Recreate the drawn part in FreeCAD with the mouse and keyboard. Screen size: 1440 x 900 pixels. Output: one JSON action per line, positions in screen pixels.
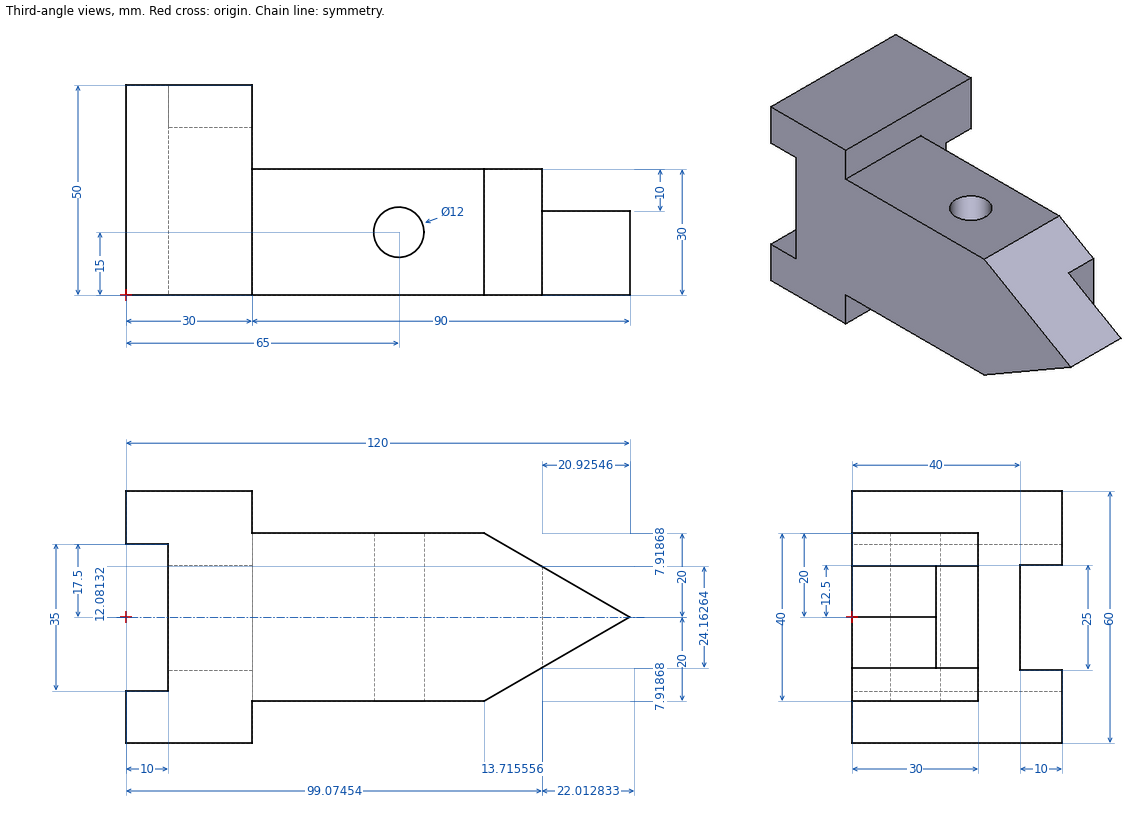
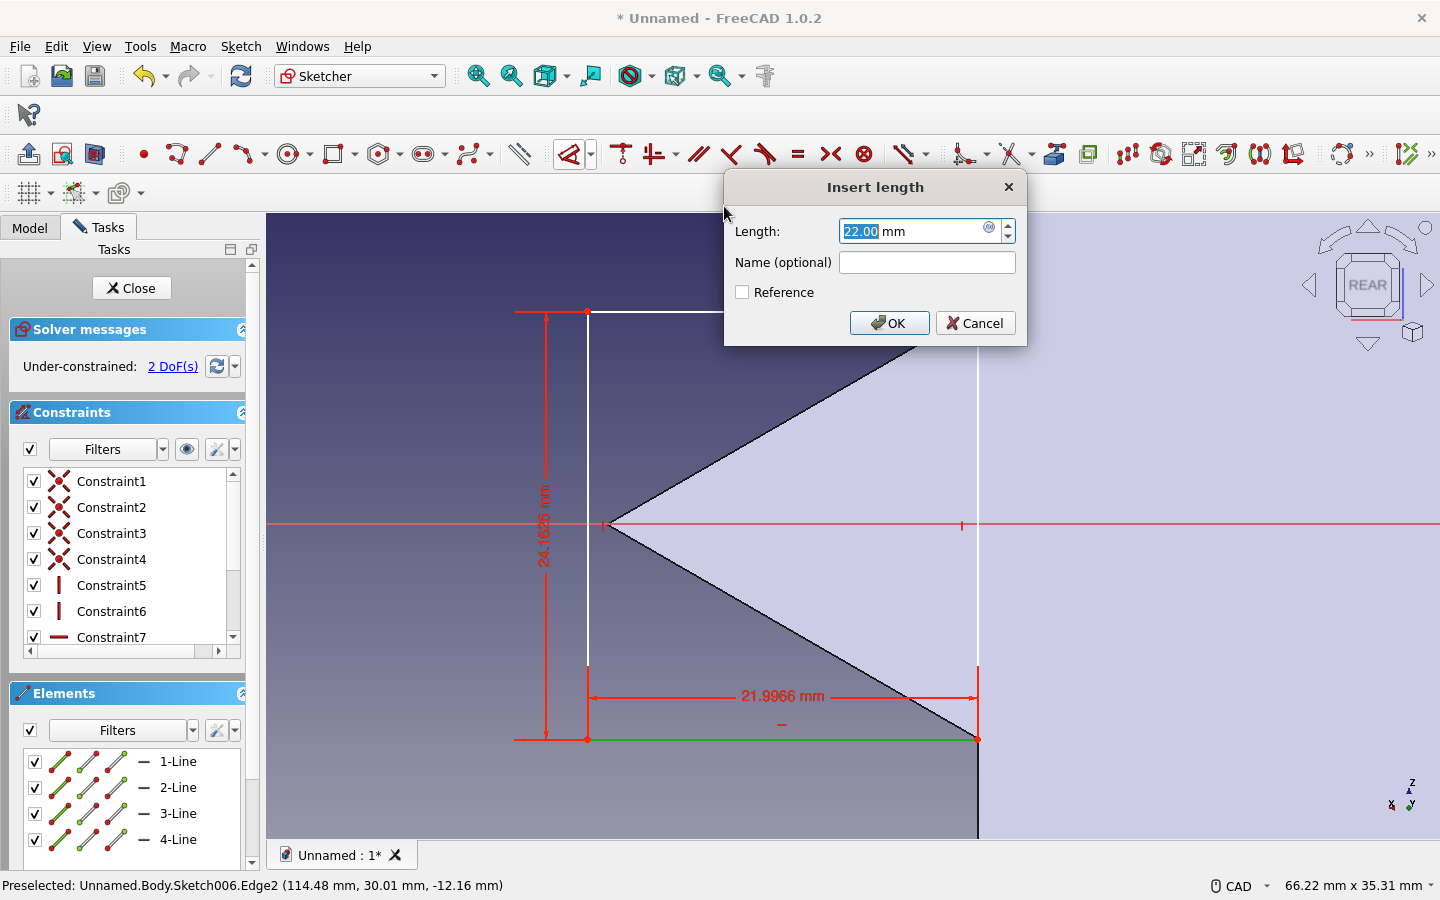
{"action": "type", "text": "22.012833"}
{"action": "key", "text": "Return"}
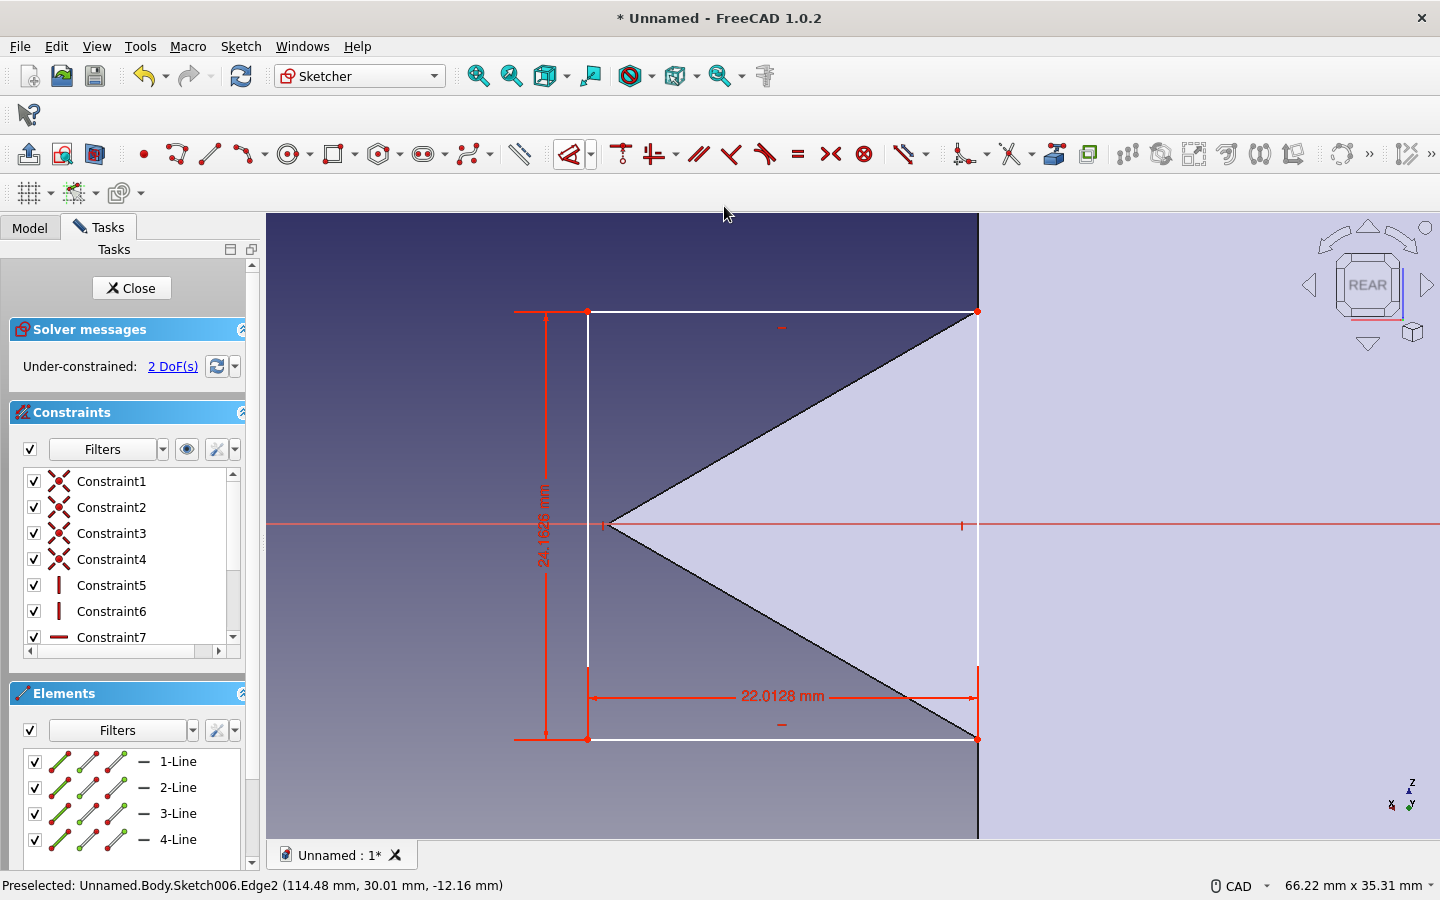
{"action": "left_click", "coordinate": [588, 312]}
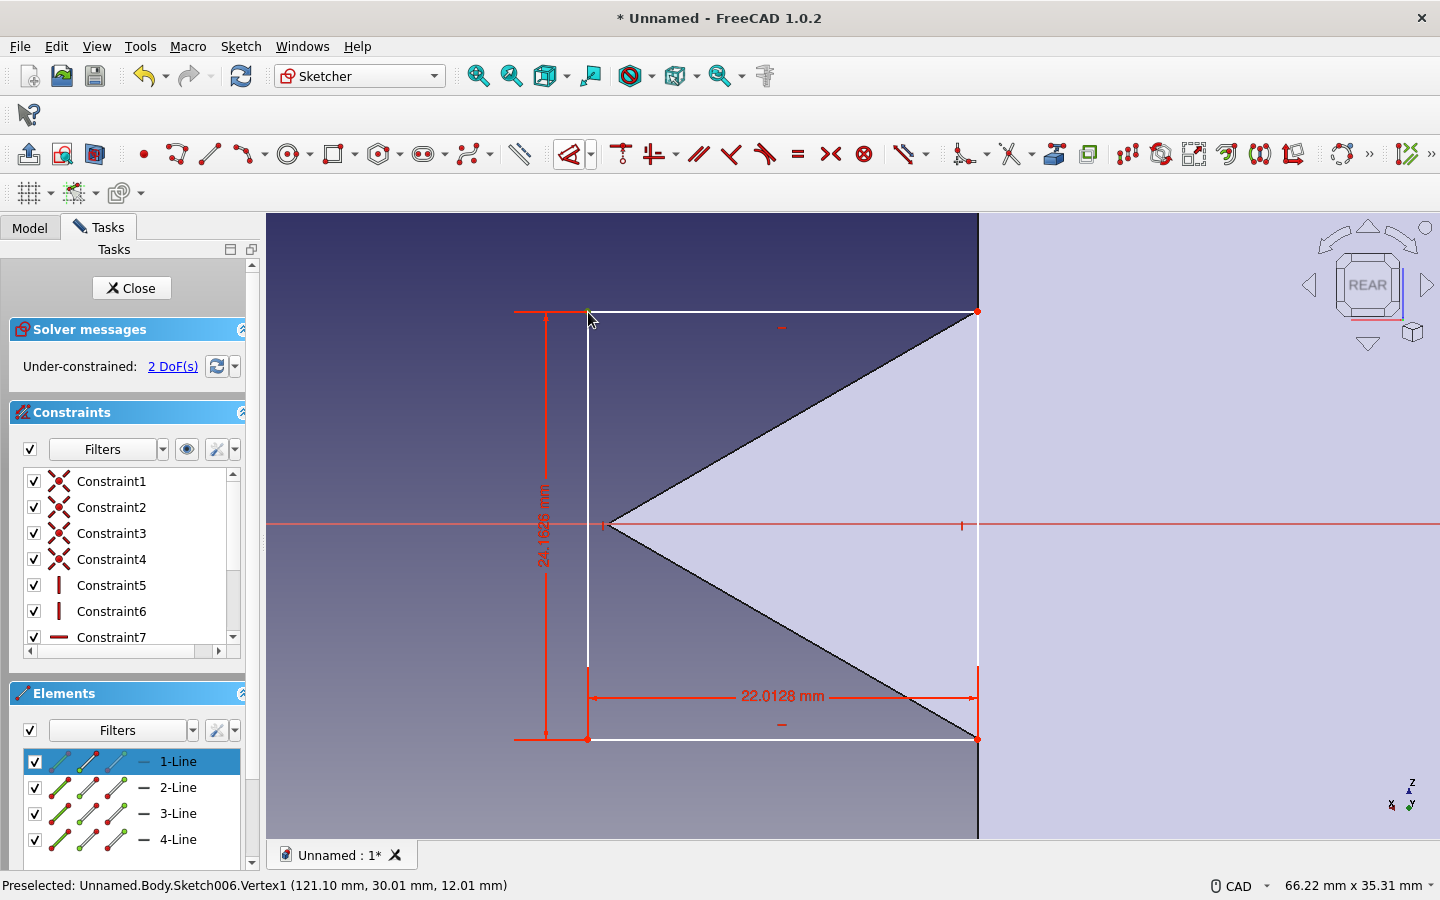
{"action": "left_click", "coordinate": [590, 154]}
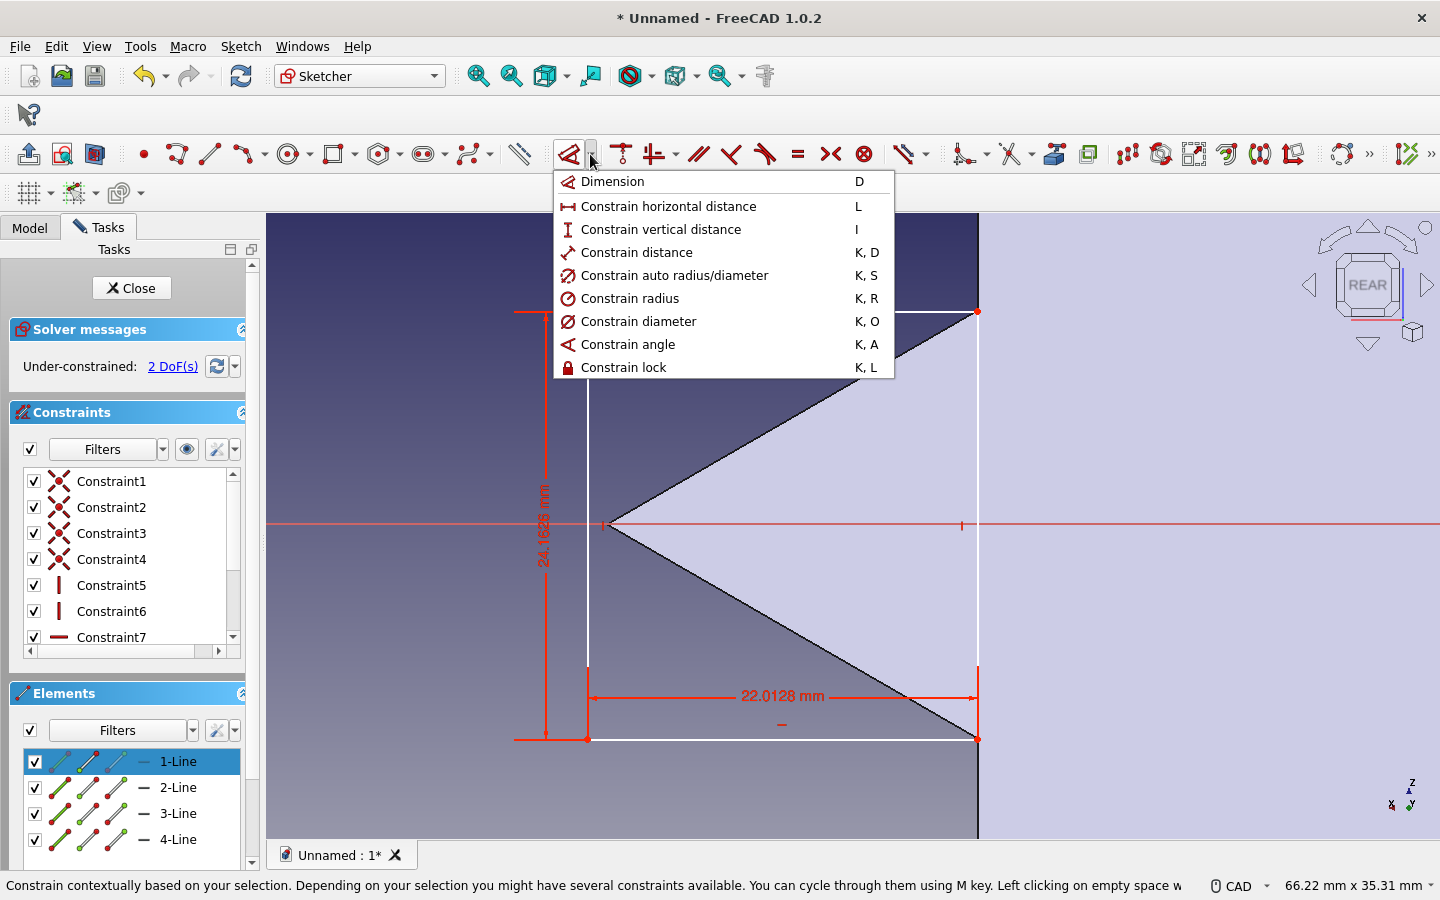
{"action": "left_click", "coordinate": [724, 230]}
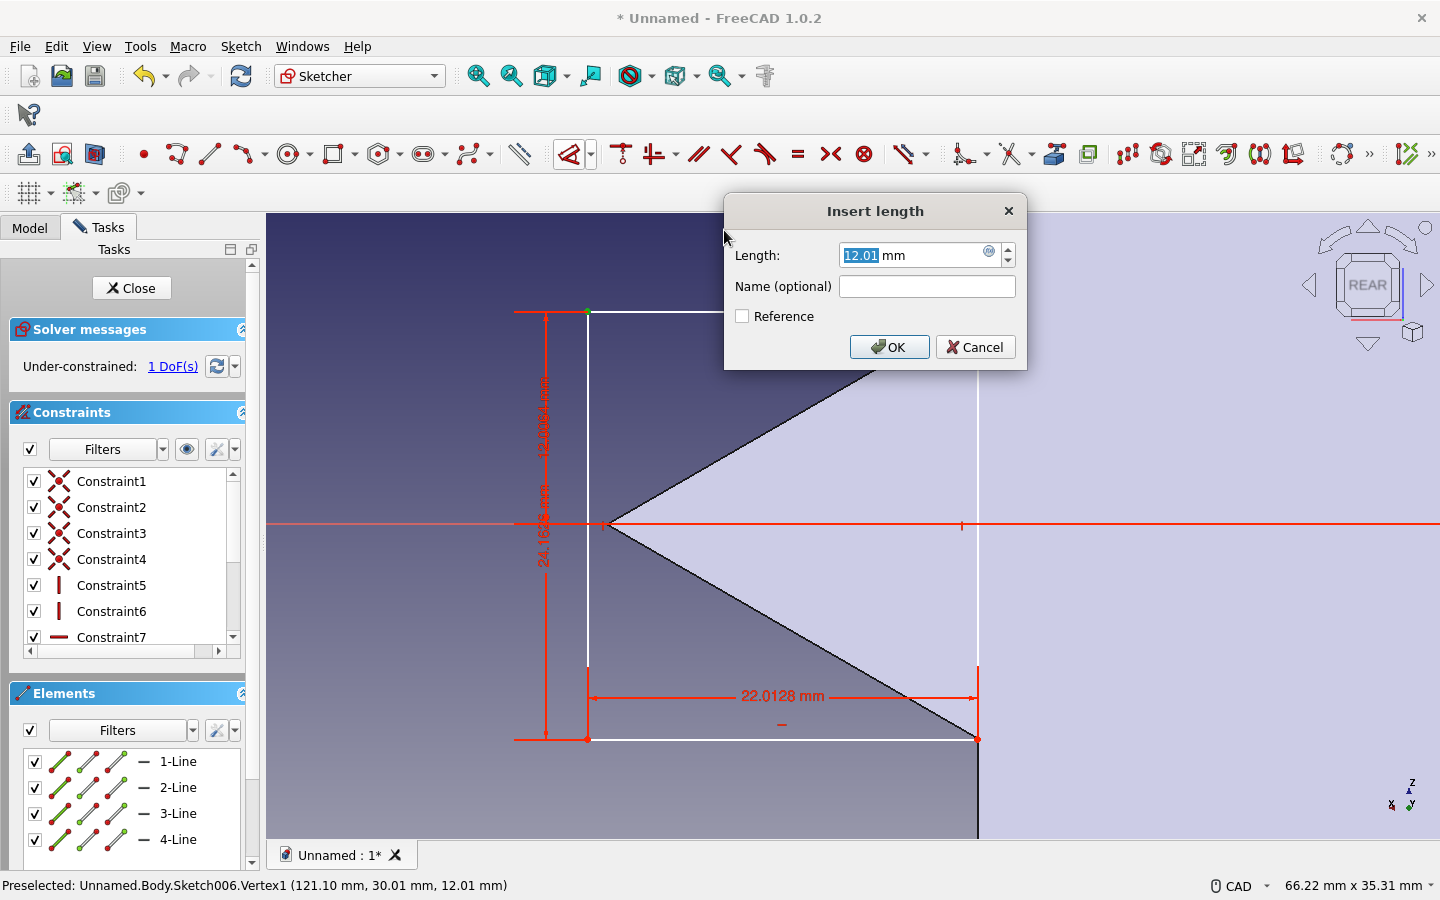
{"action": "type", "text": "12.08132"}
{"action": "key", "text": "Return"}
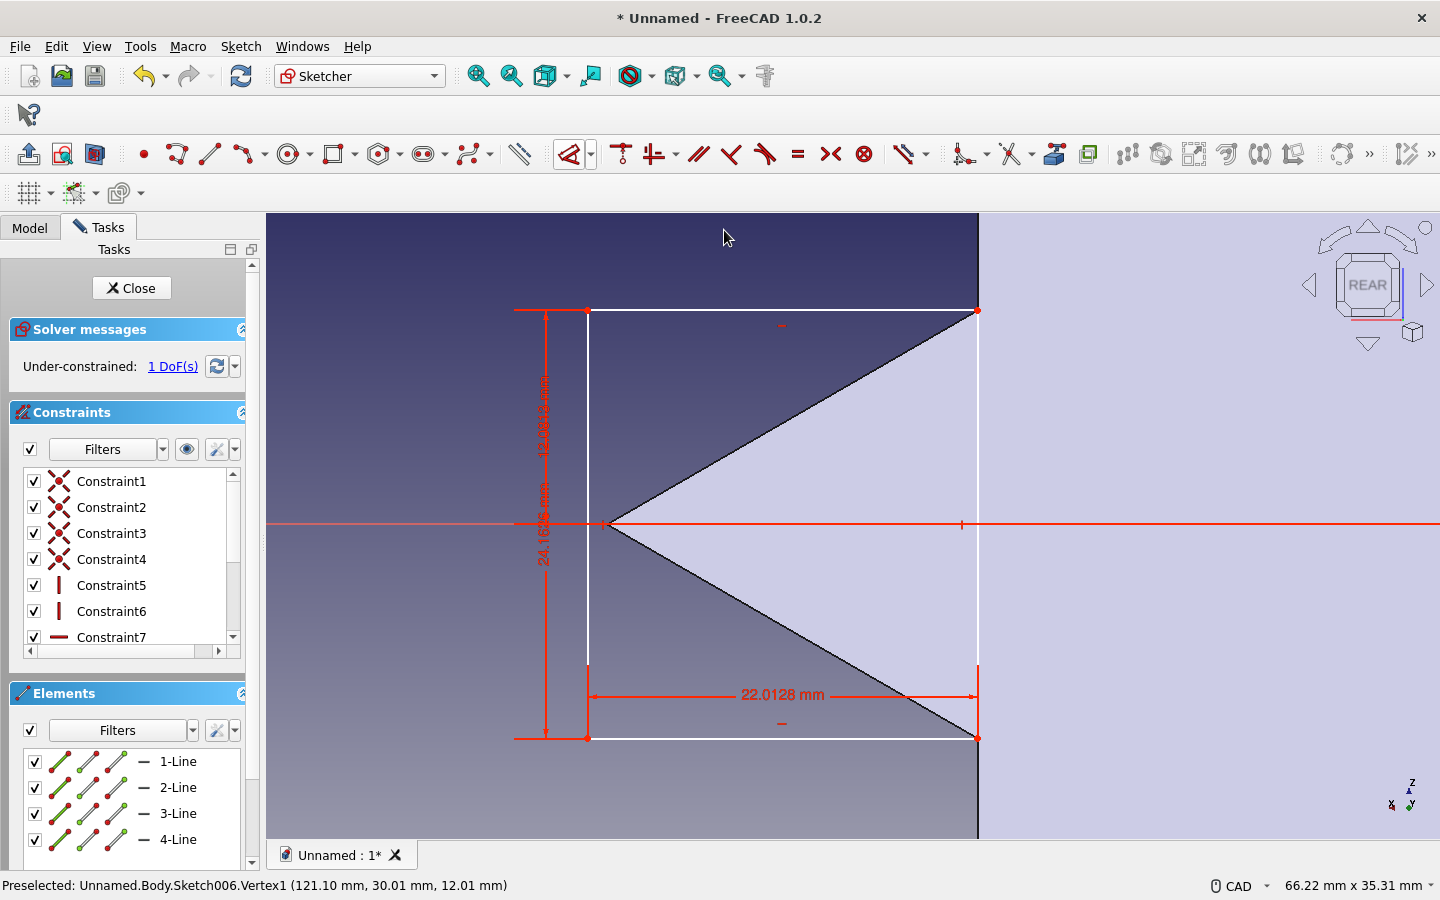
{"action": "left_click", "coordinate": [978, 739]}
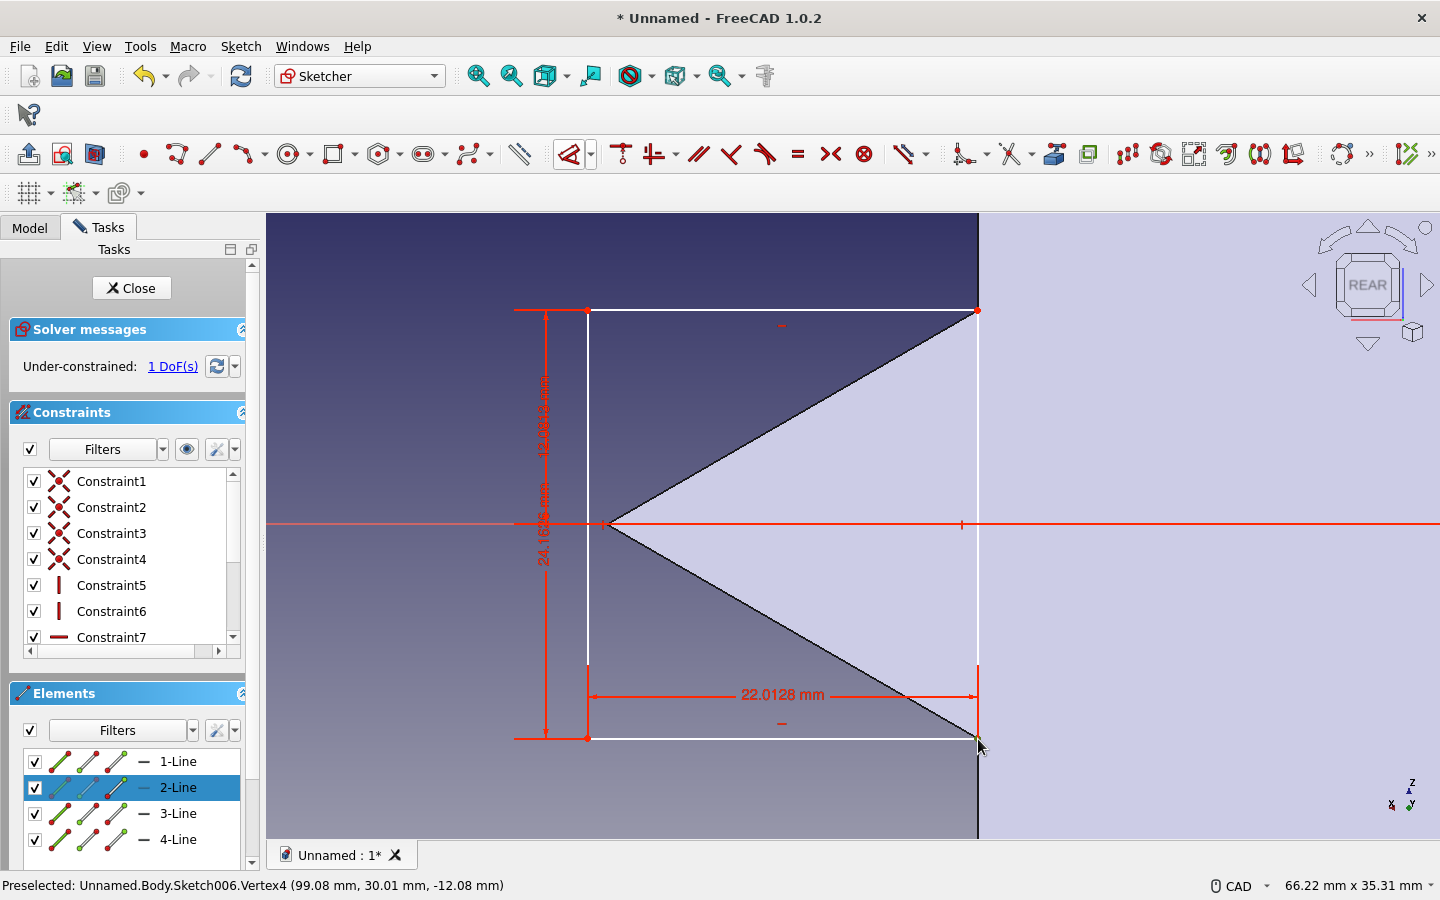
{"action": "left_click", "coordinate": [590, 154]}